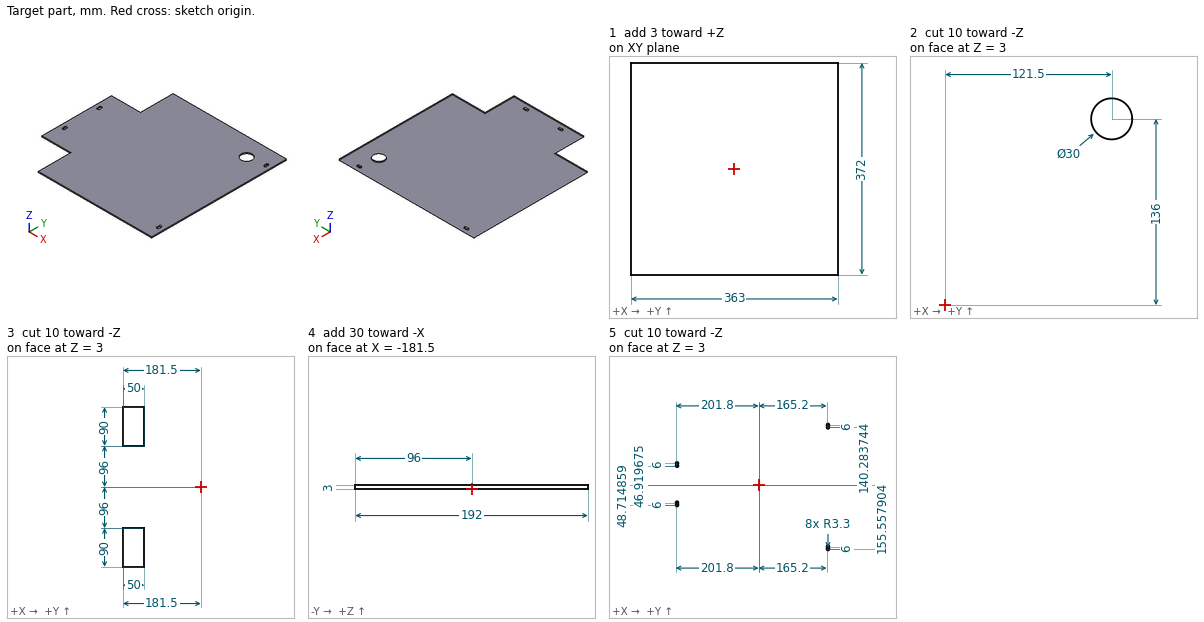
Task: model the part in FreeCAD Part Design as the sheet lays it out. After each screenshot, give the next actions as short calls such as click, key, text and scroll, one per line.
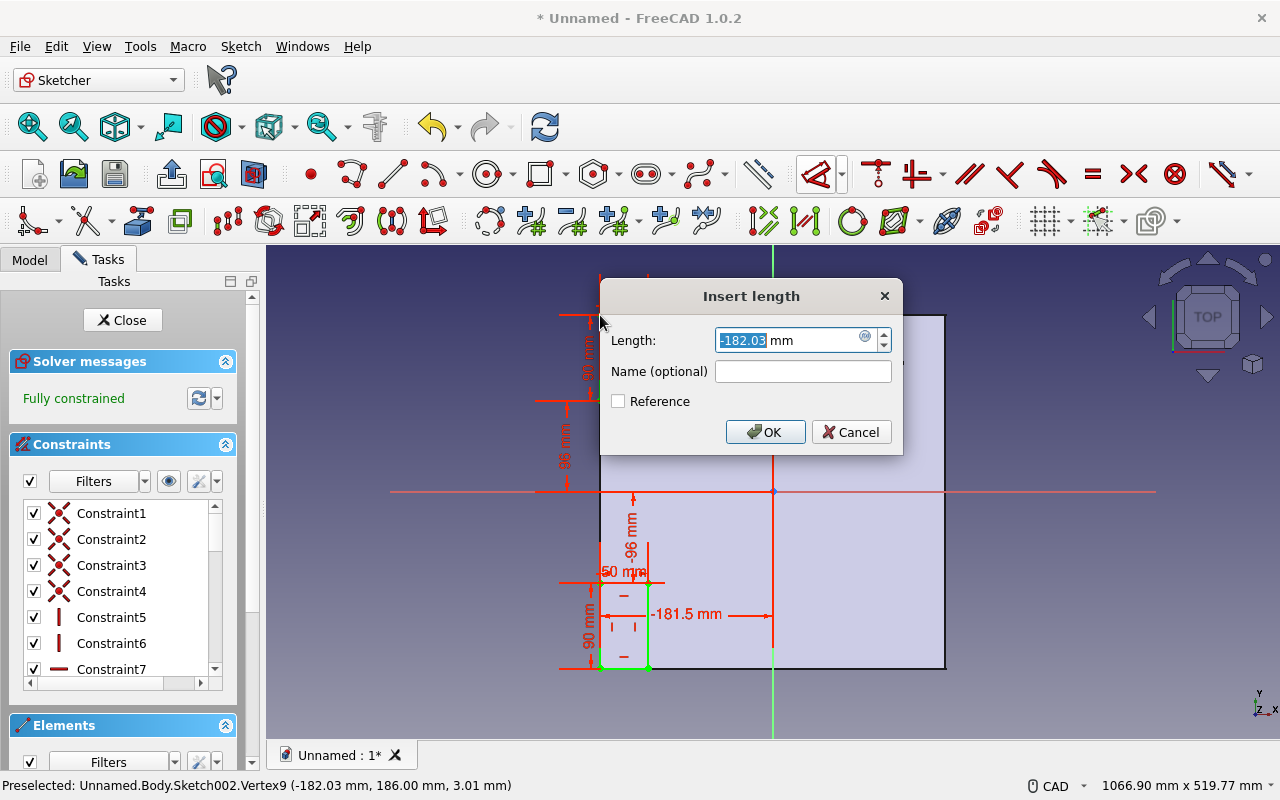
text(-181.5)
key(Return)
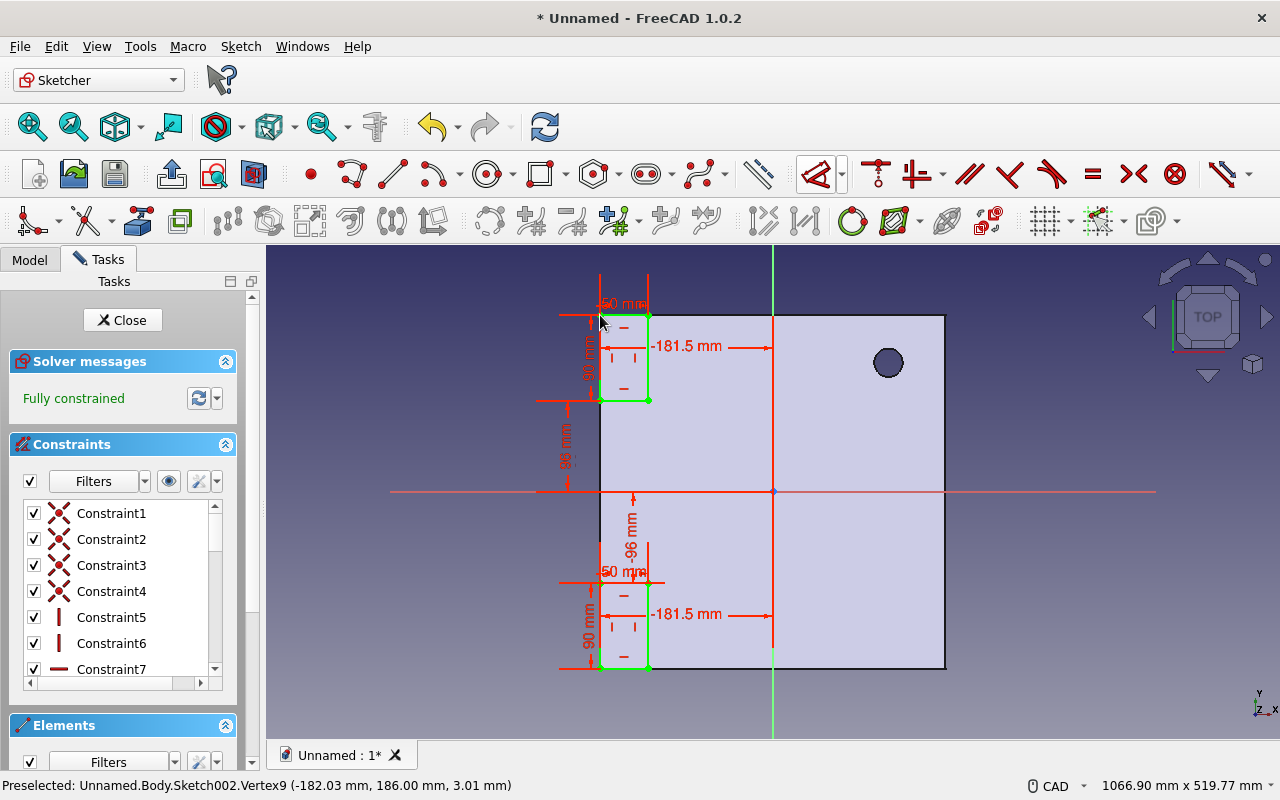
click(123, 320)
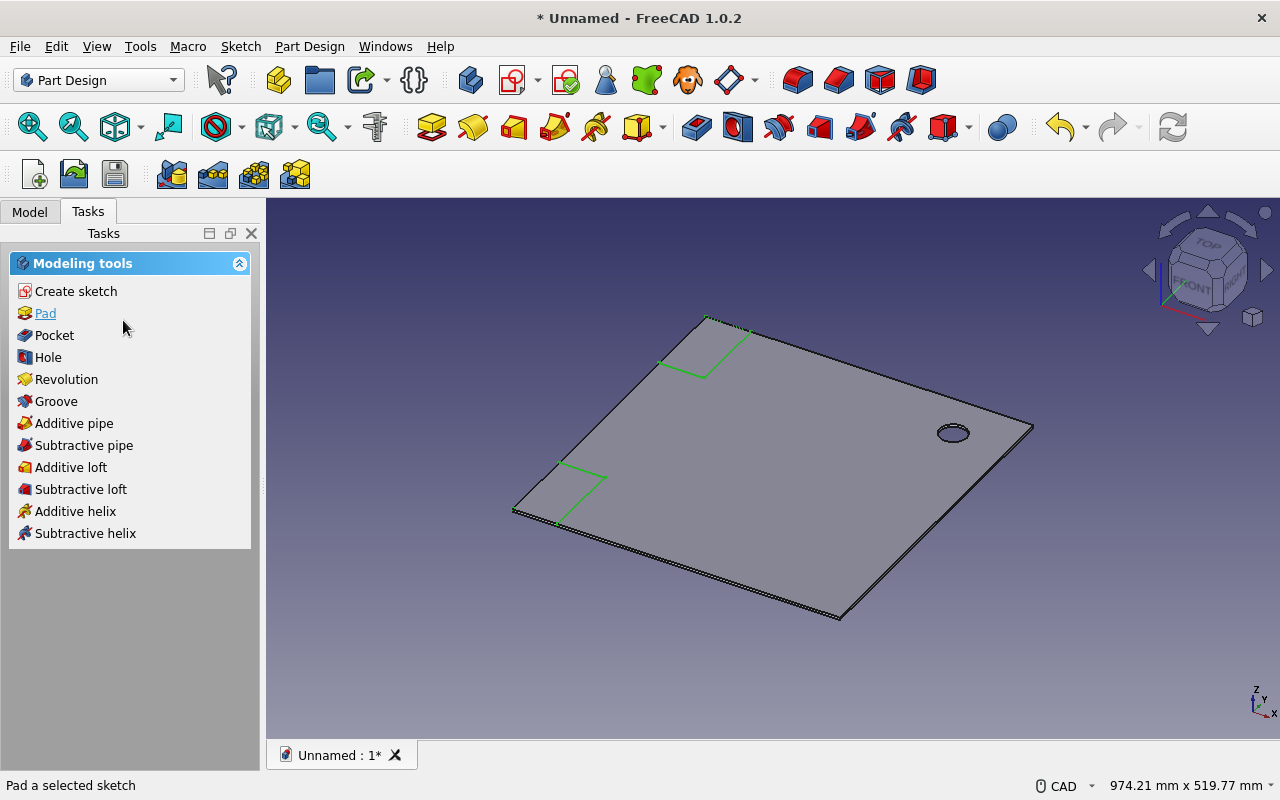
click(697, 128)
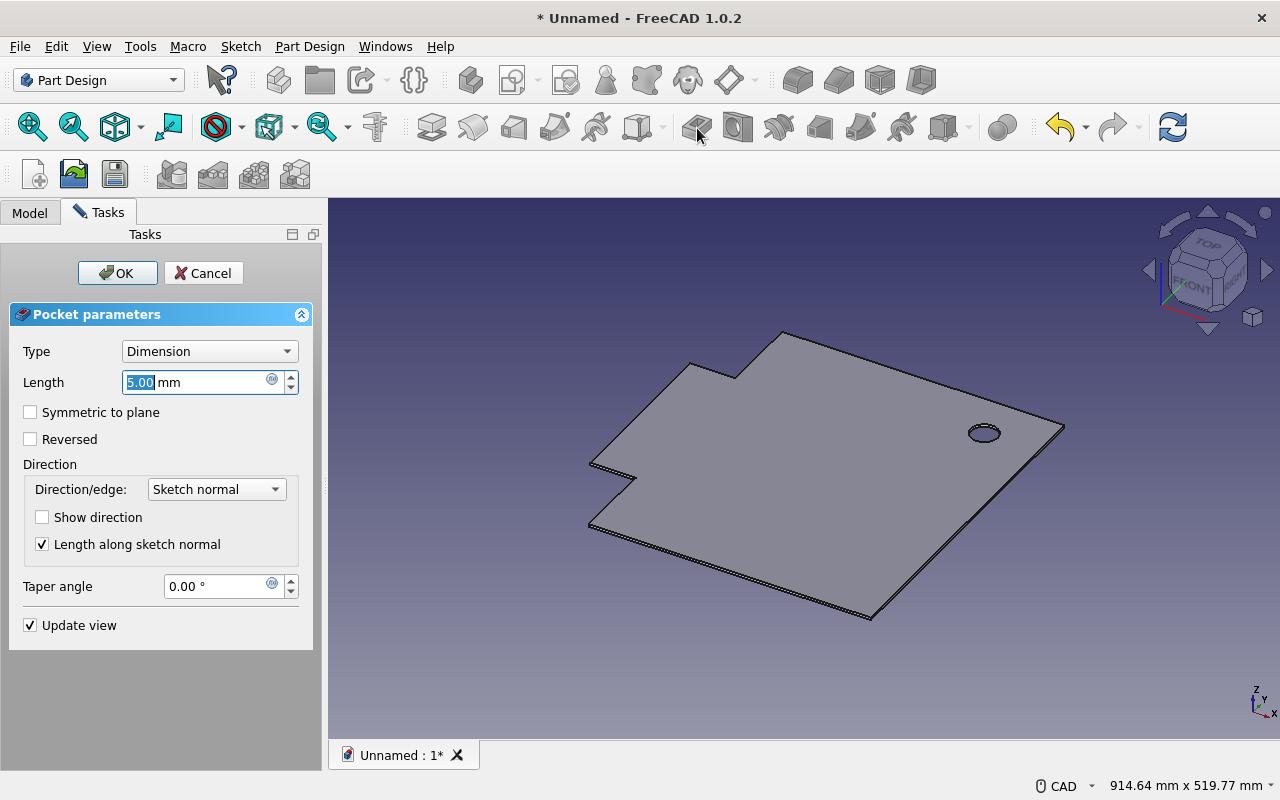
text(10)
key(Tab)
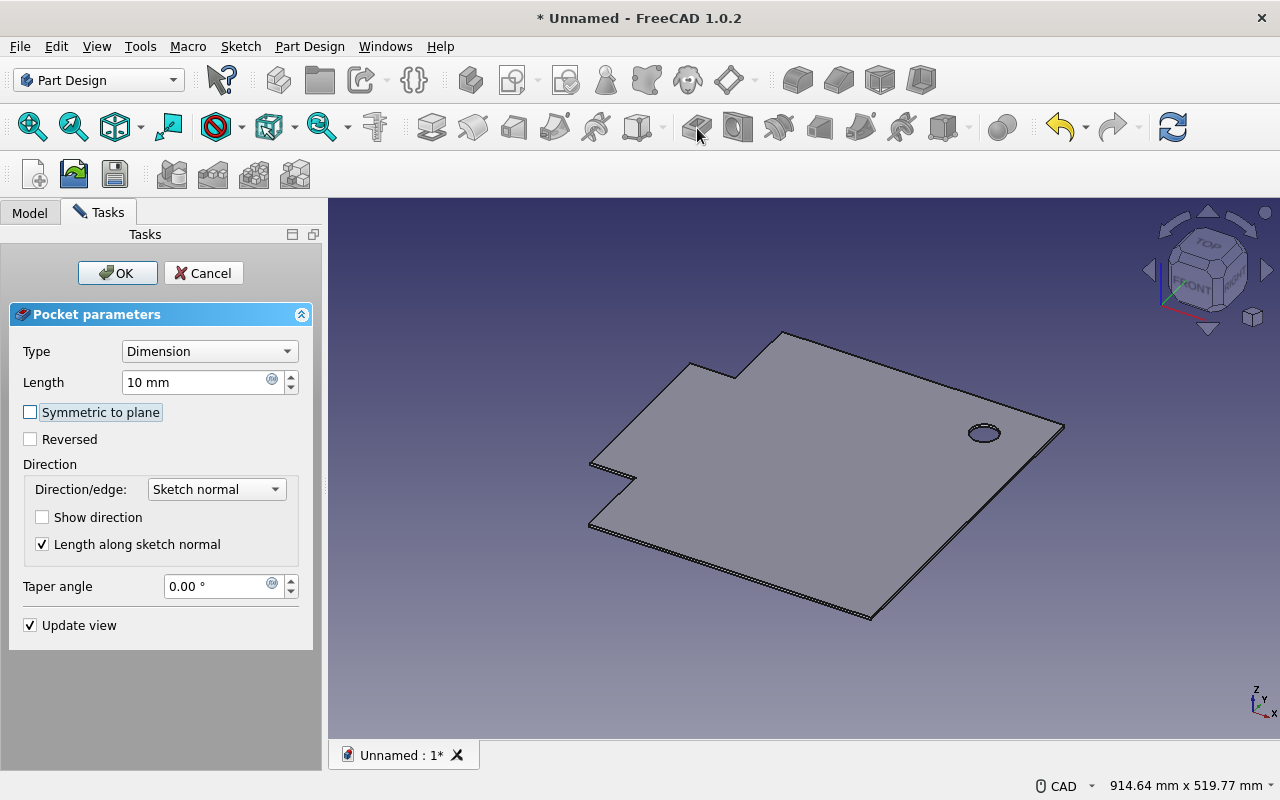
click(118, 273)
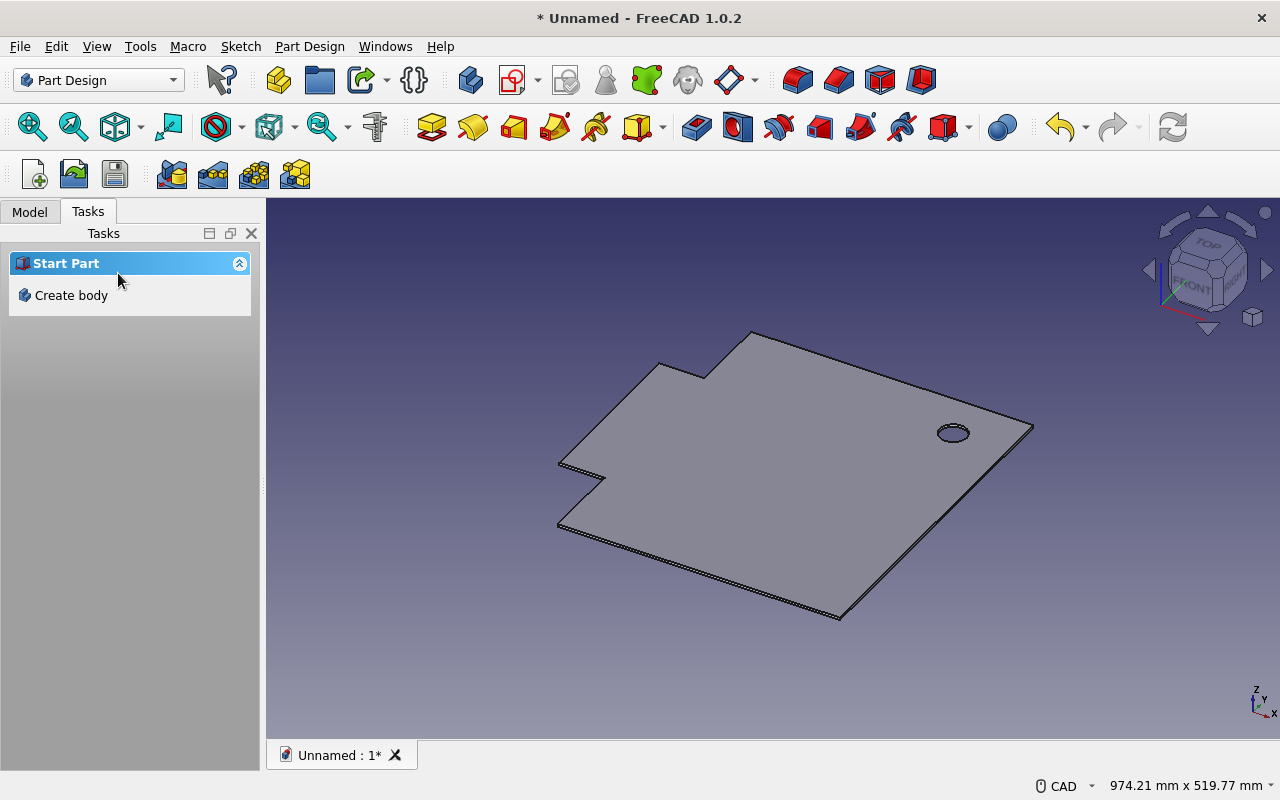
key(6)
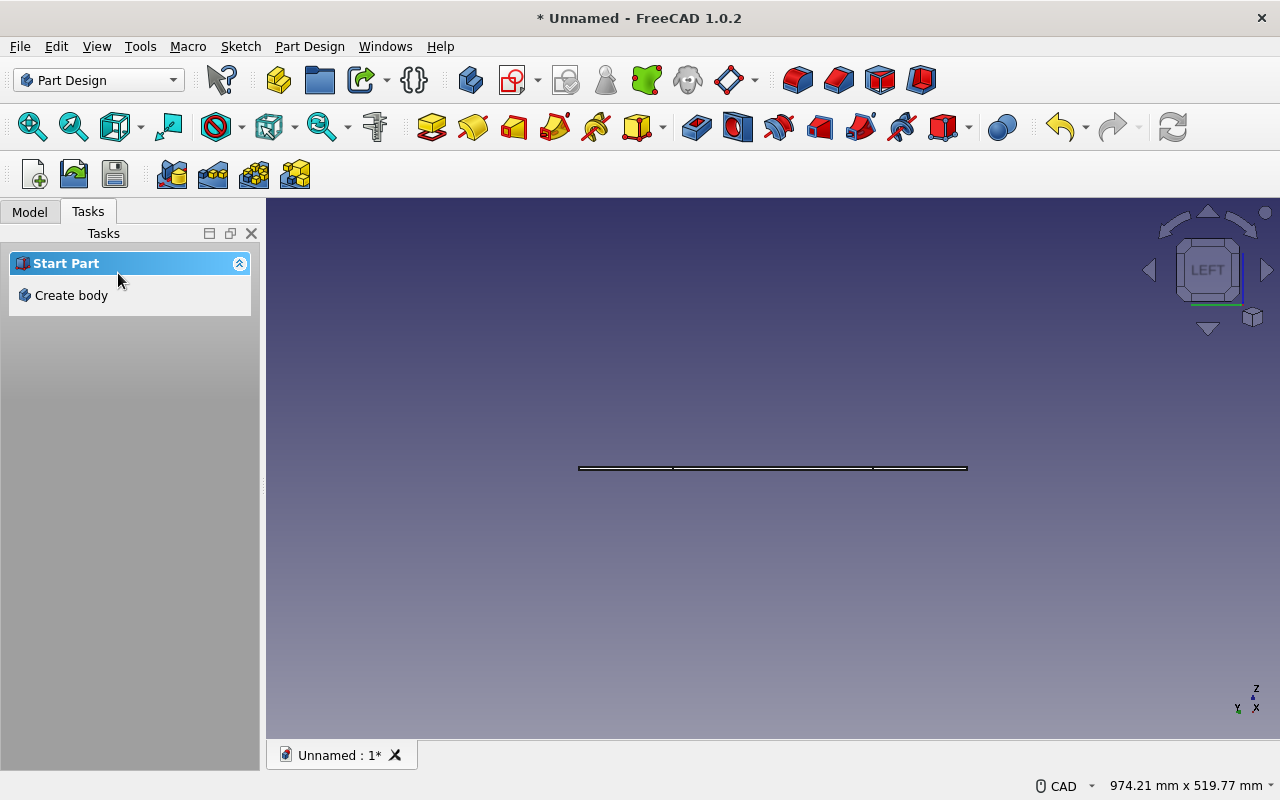
click(33, 128)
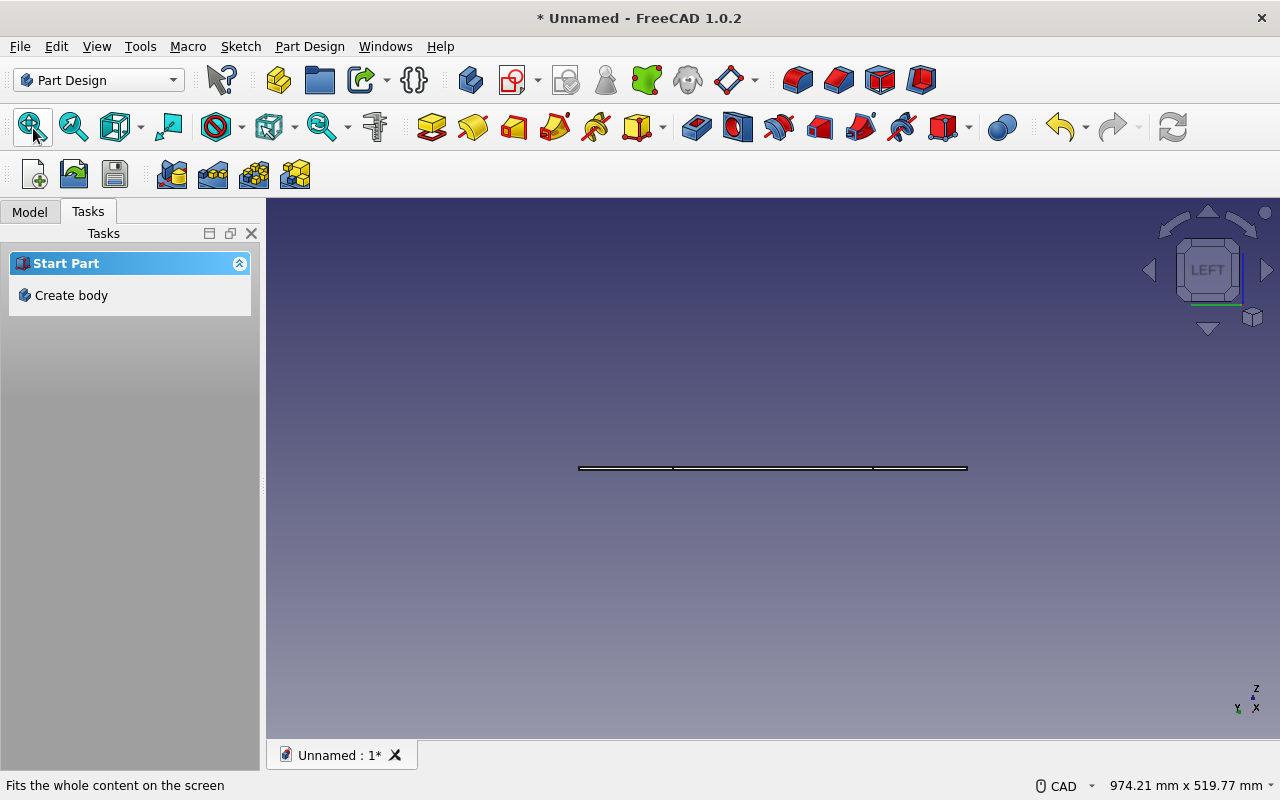
scroll(687, 467, up, 11)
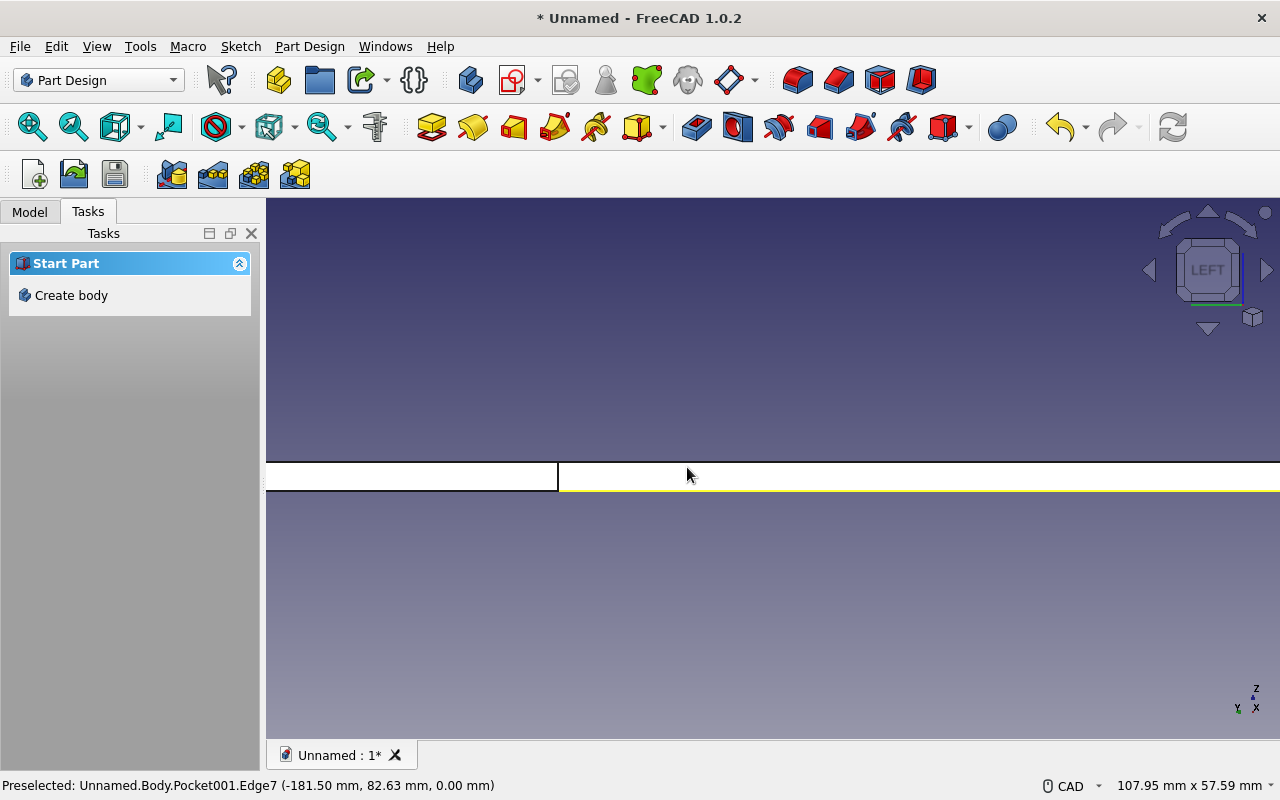
click(687, 476)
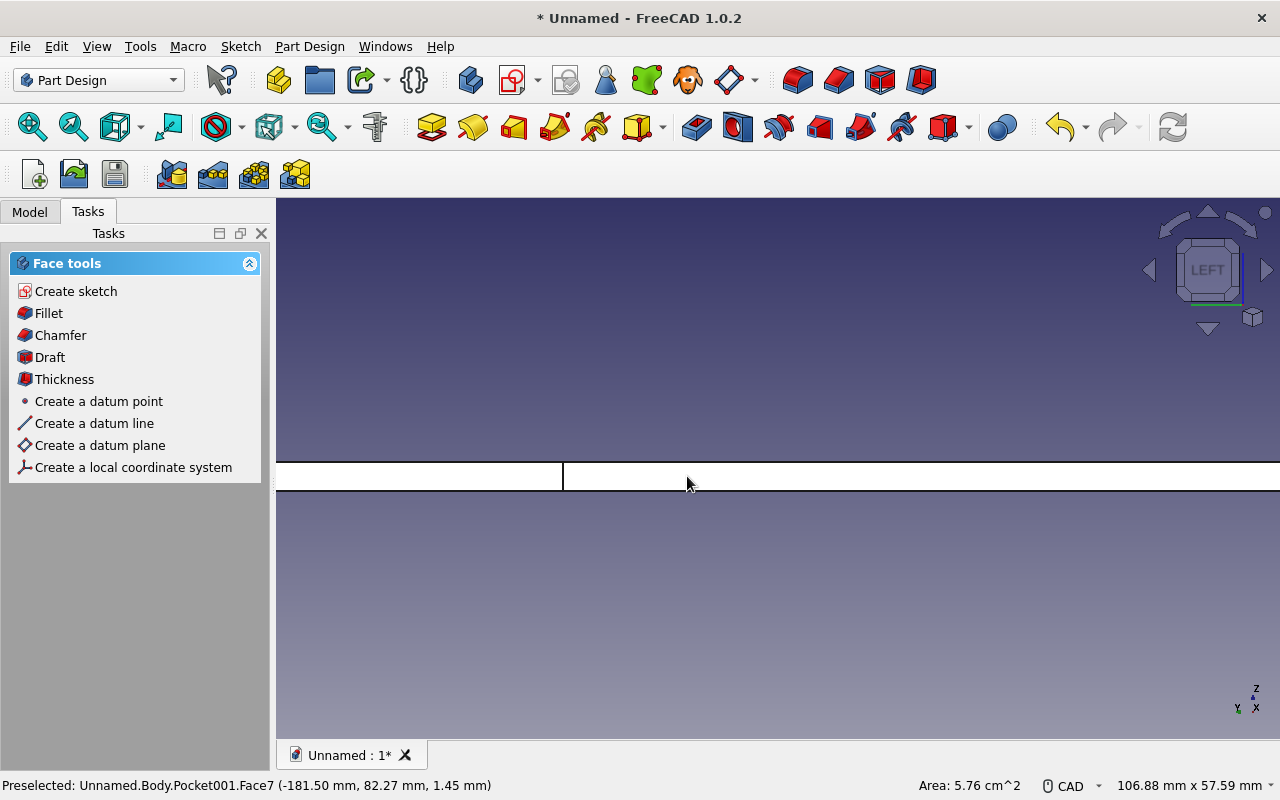
click(512, 80)